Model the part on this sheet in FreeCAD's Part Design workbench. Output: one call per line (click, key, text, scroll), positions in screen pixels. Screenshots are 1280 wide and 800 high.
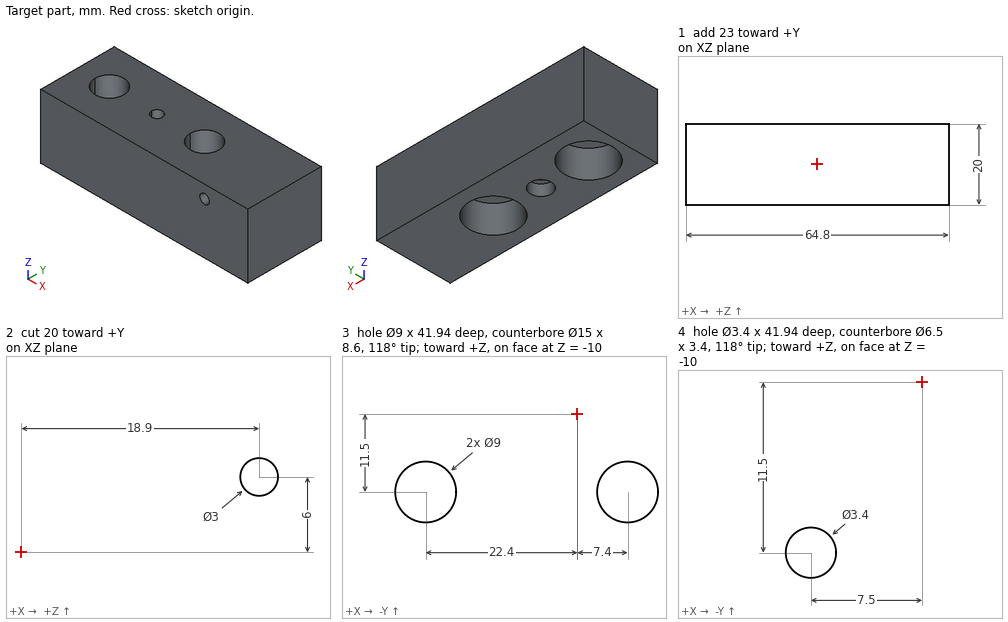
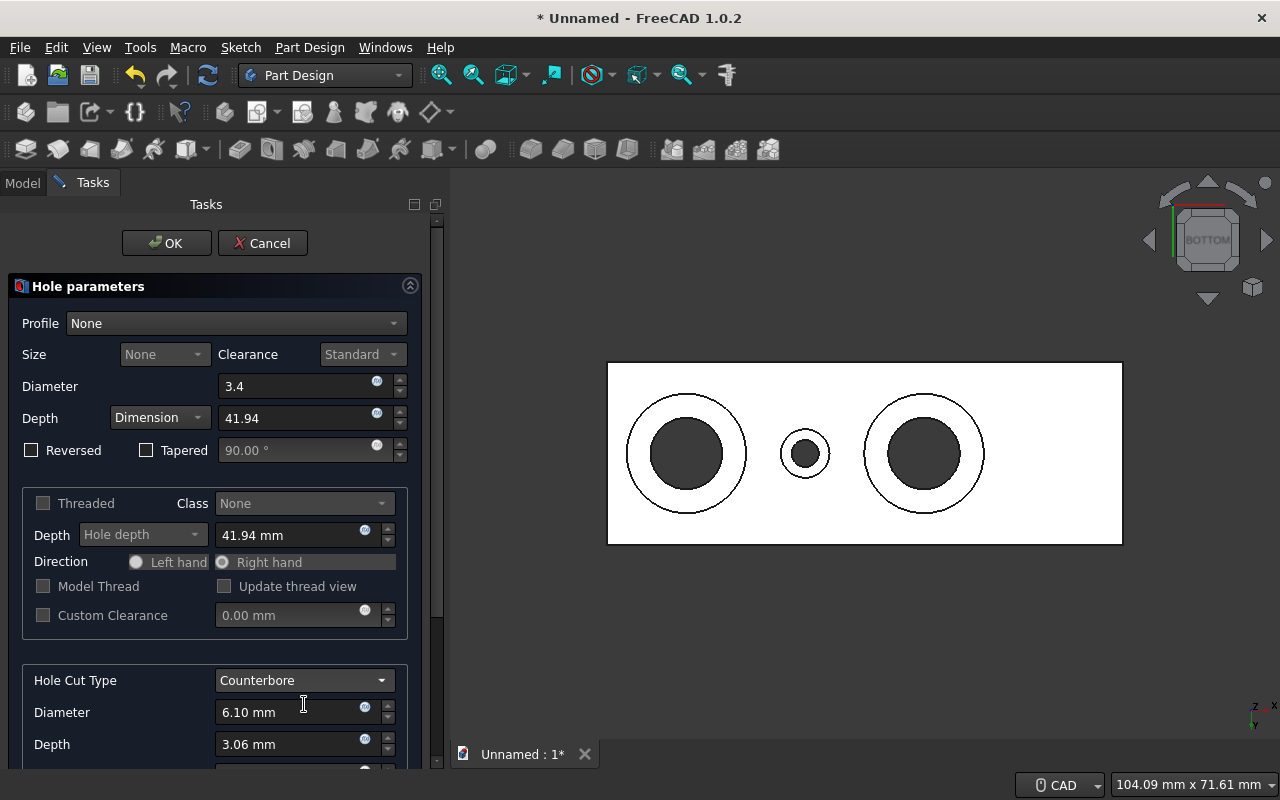
triple_click(298, 712)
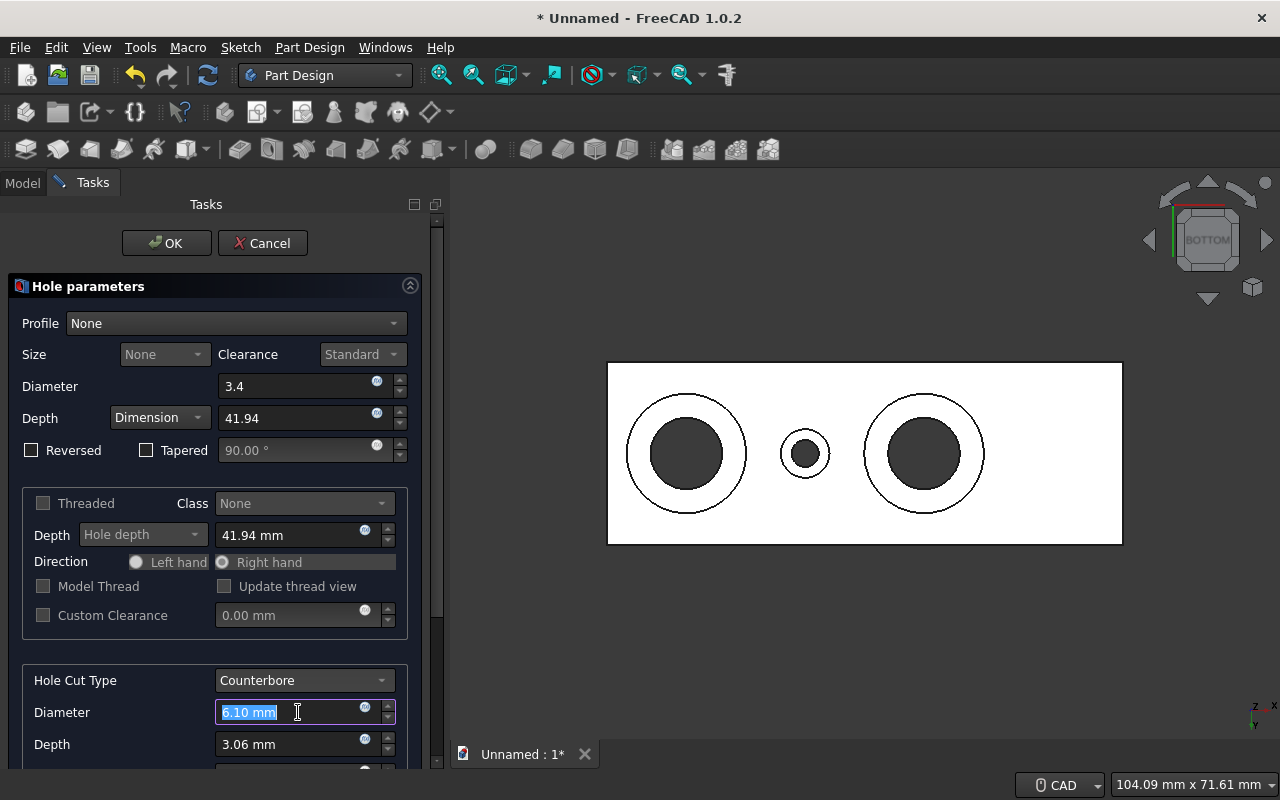
text(6.5)
key(Tab)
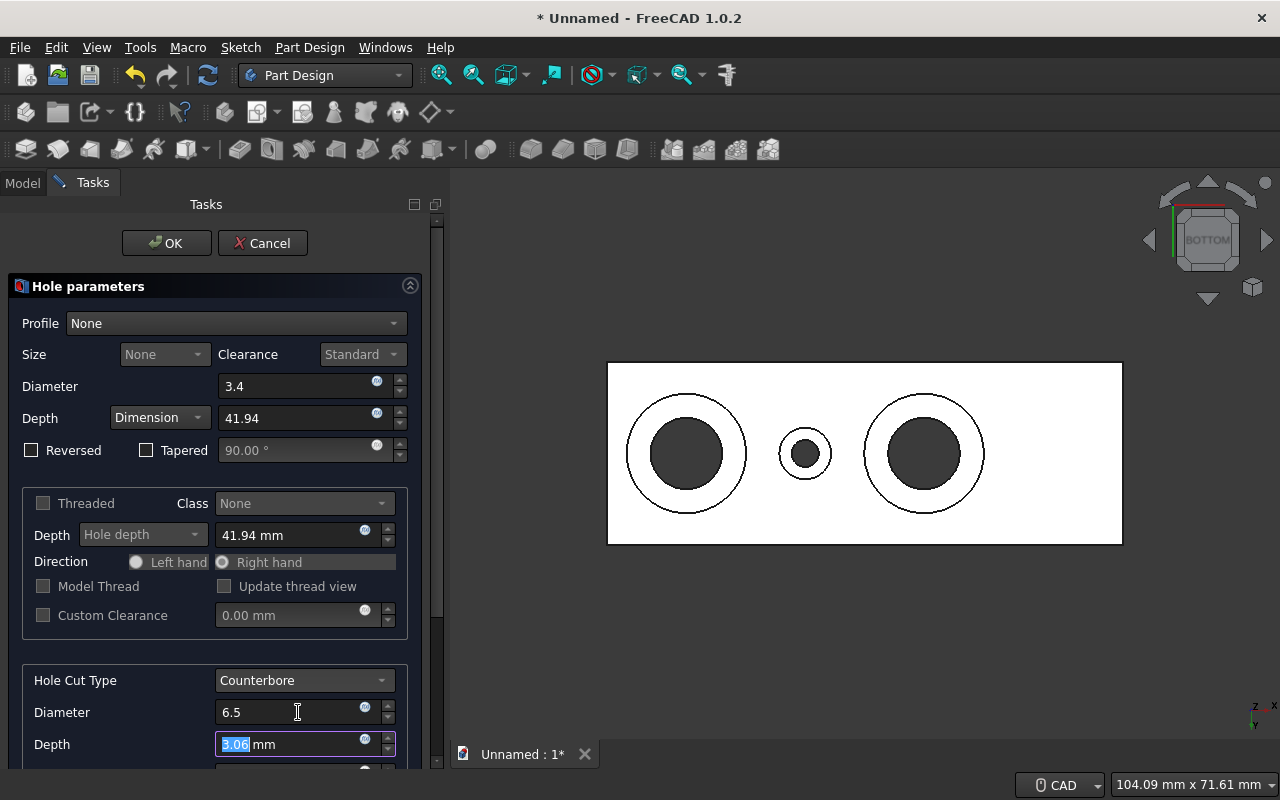
text(3.4)
key(Tab)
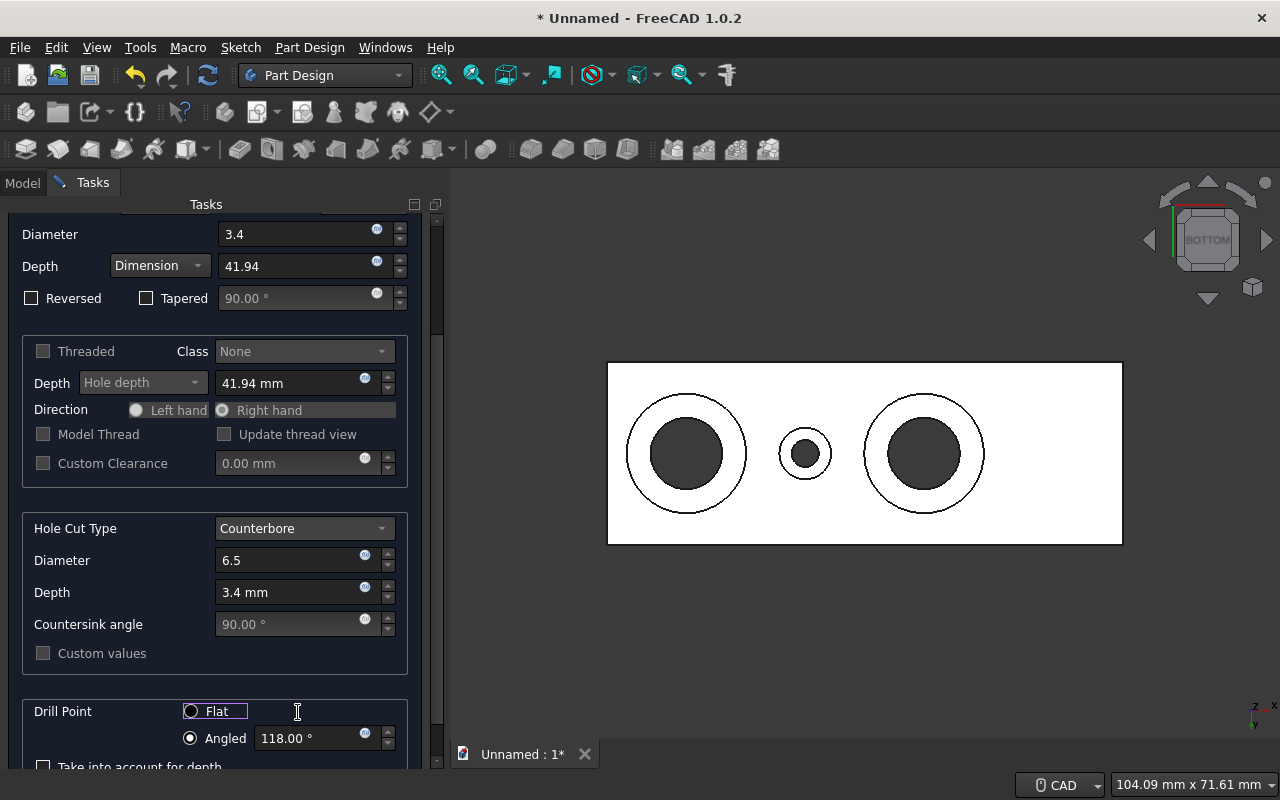
scroll(437, 491, up, 4)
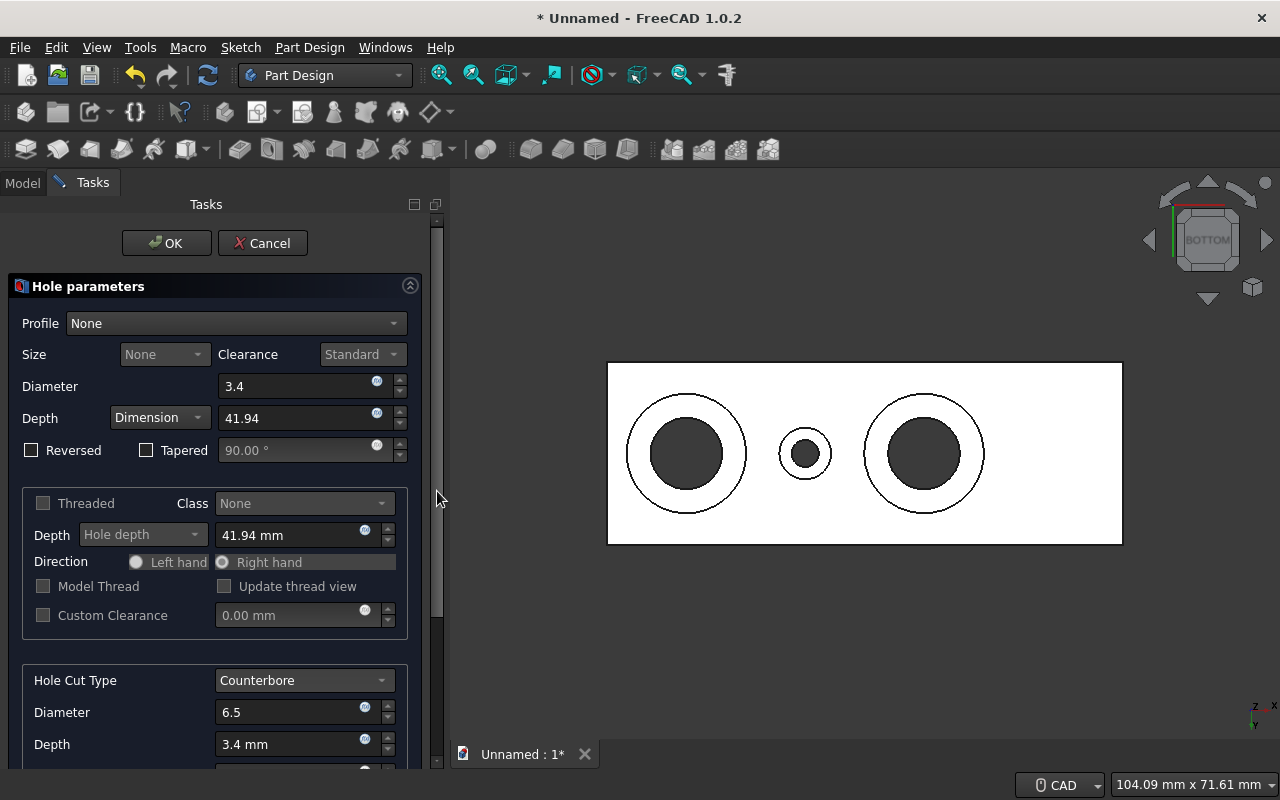
click(167, 243)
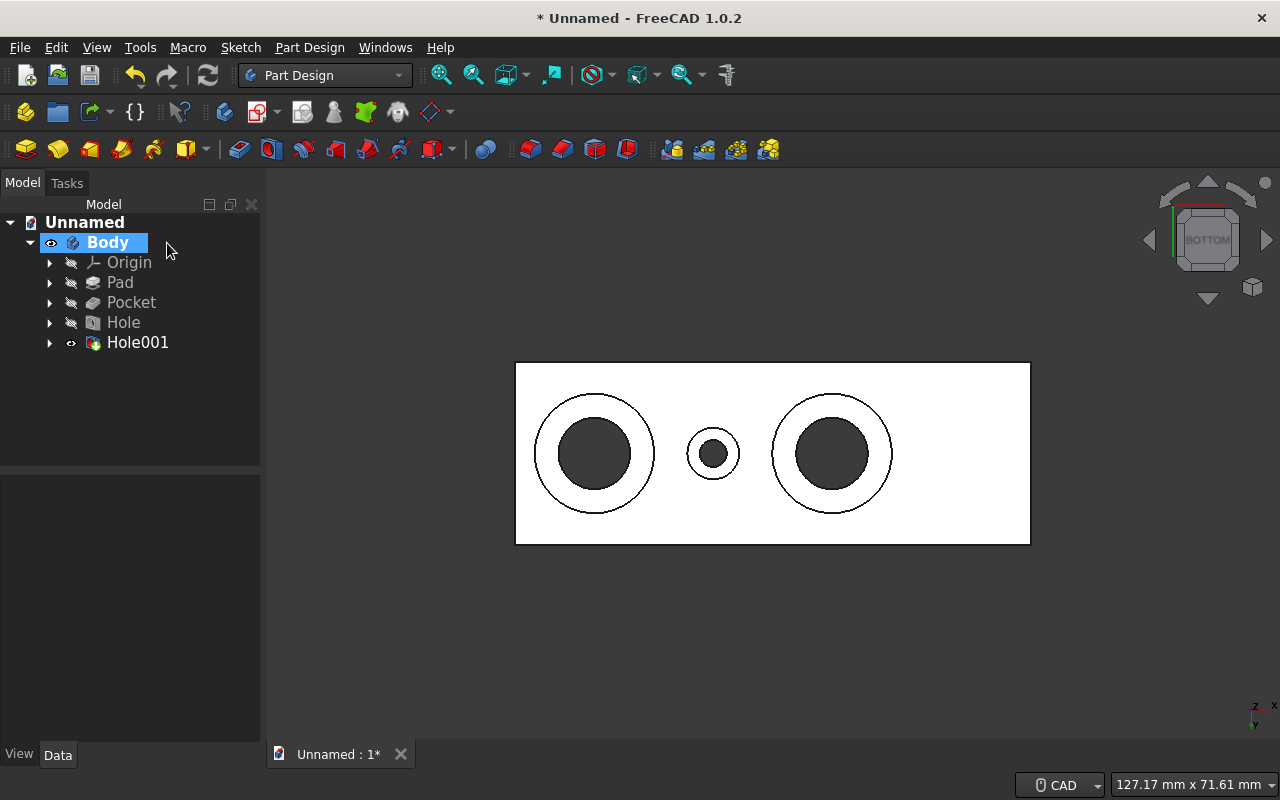
key(0)